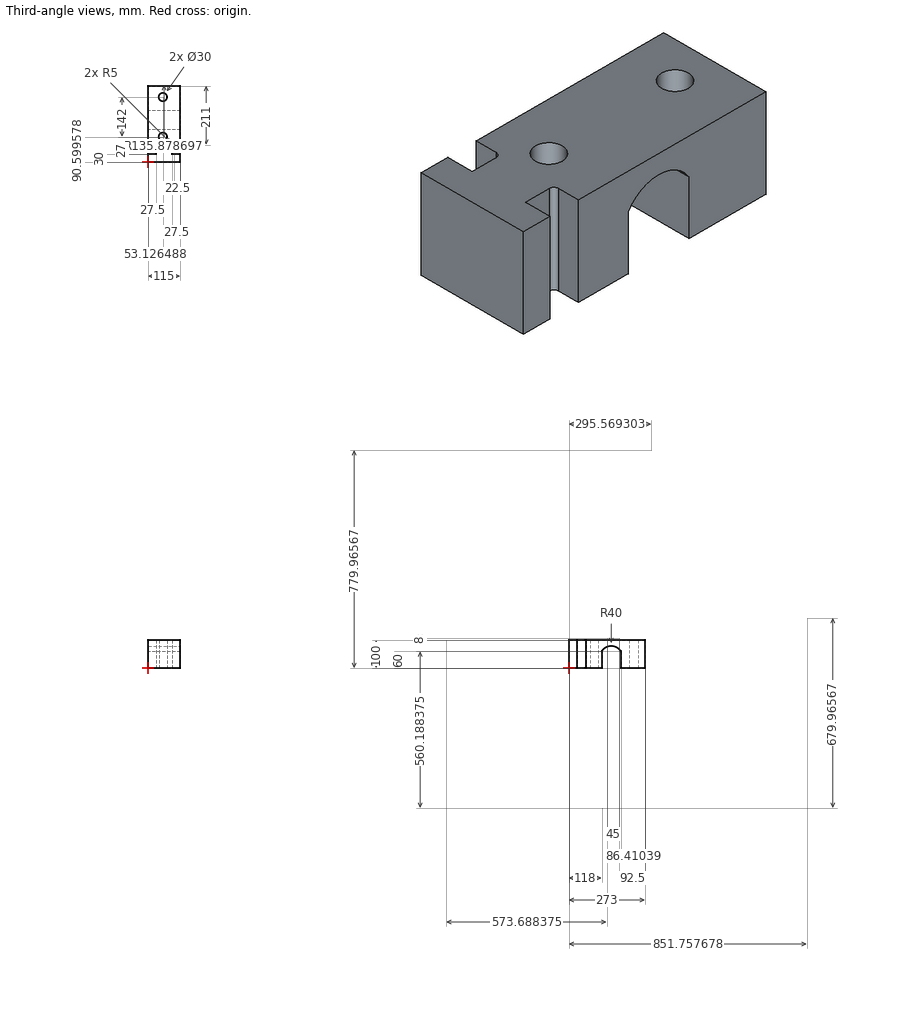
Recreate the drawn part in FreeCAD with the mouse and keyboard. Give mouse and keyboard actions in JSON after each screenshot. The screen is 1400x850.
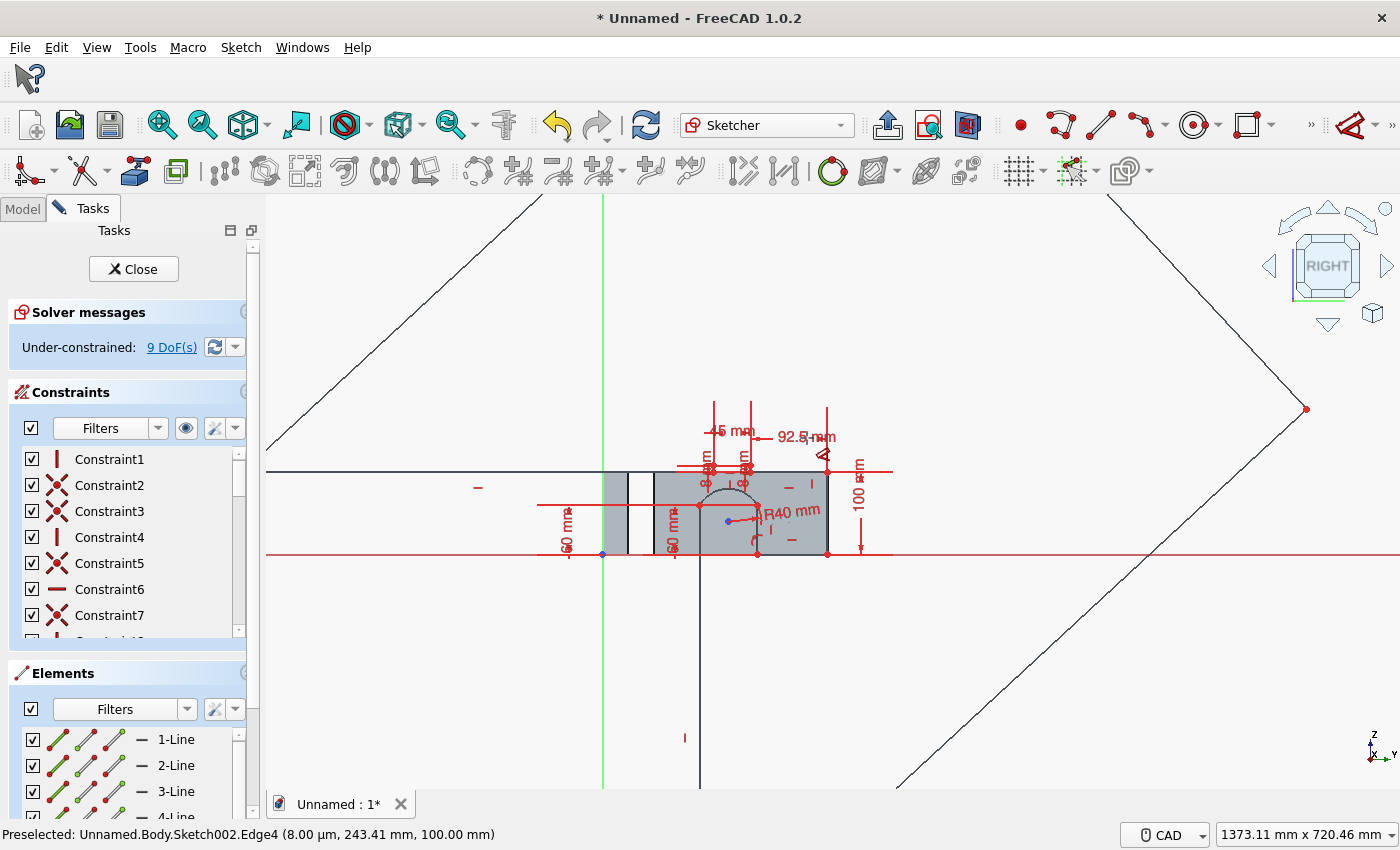
{"action": "left_click", "coordinate": [827, 555]}
{"action": "left_click", "coordinate": [715, 589]}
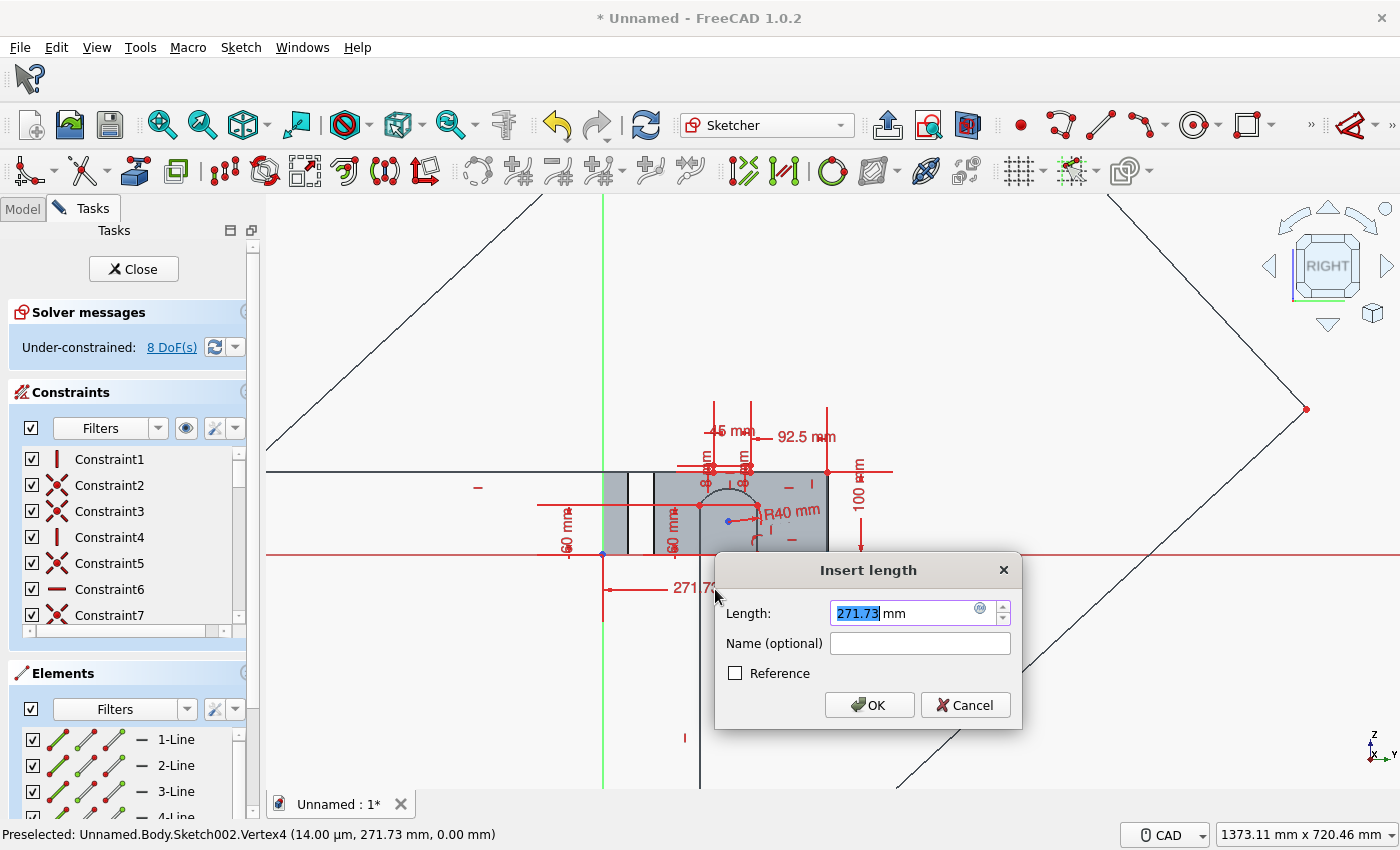
{"action": "type", "text": "273"}
{"action": "key", "text": "Return"}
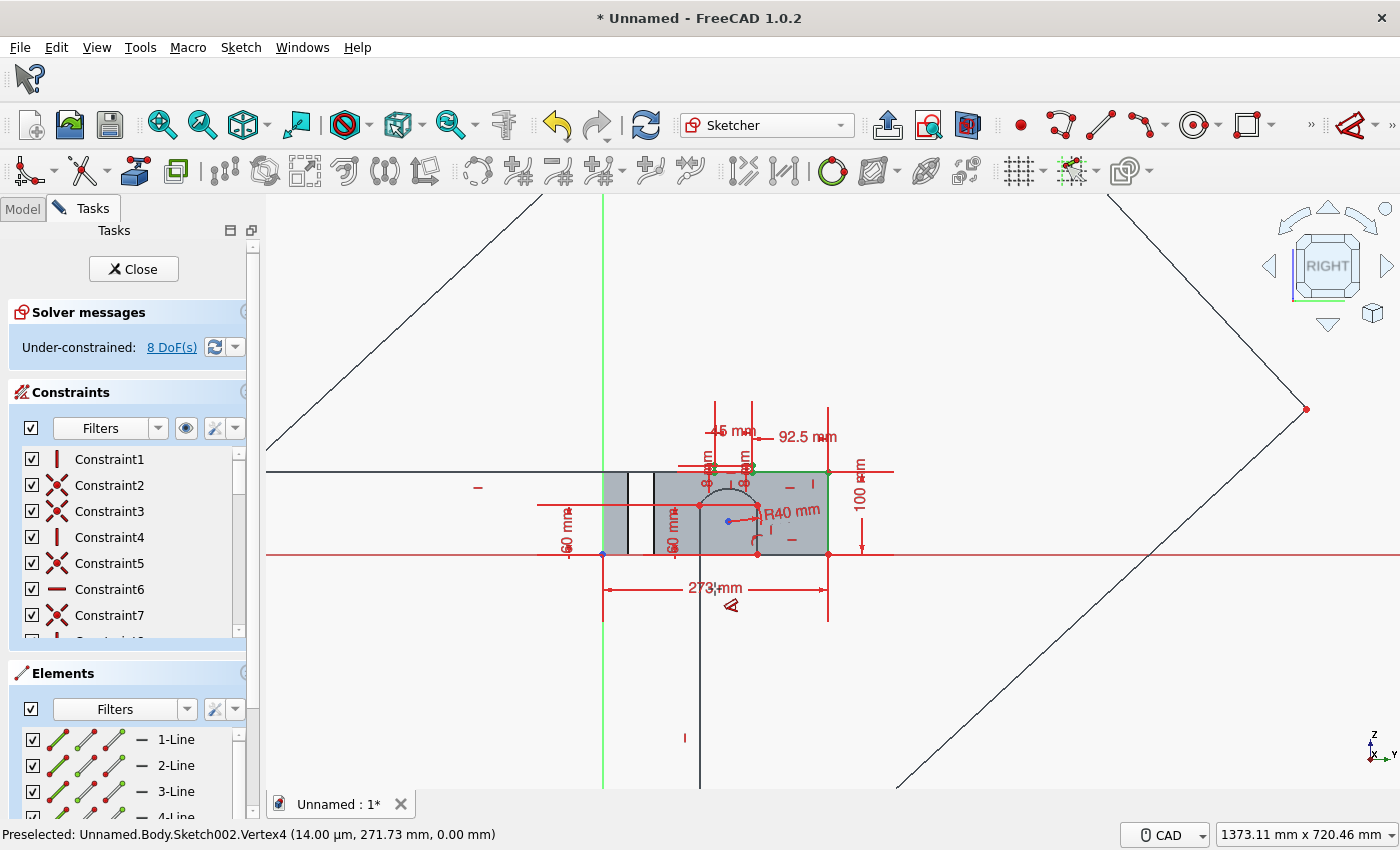
{"action": "scroll", "coordinate": [759, 522], "scroll_direction": "down", "scroll_amount": 5}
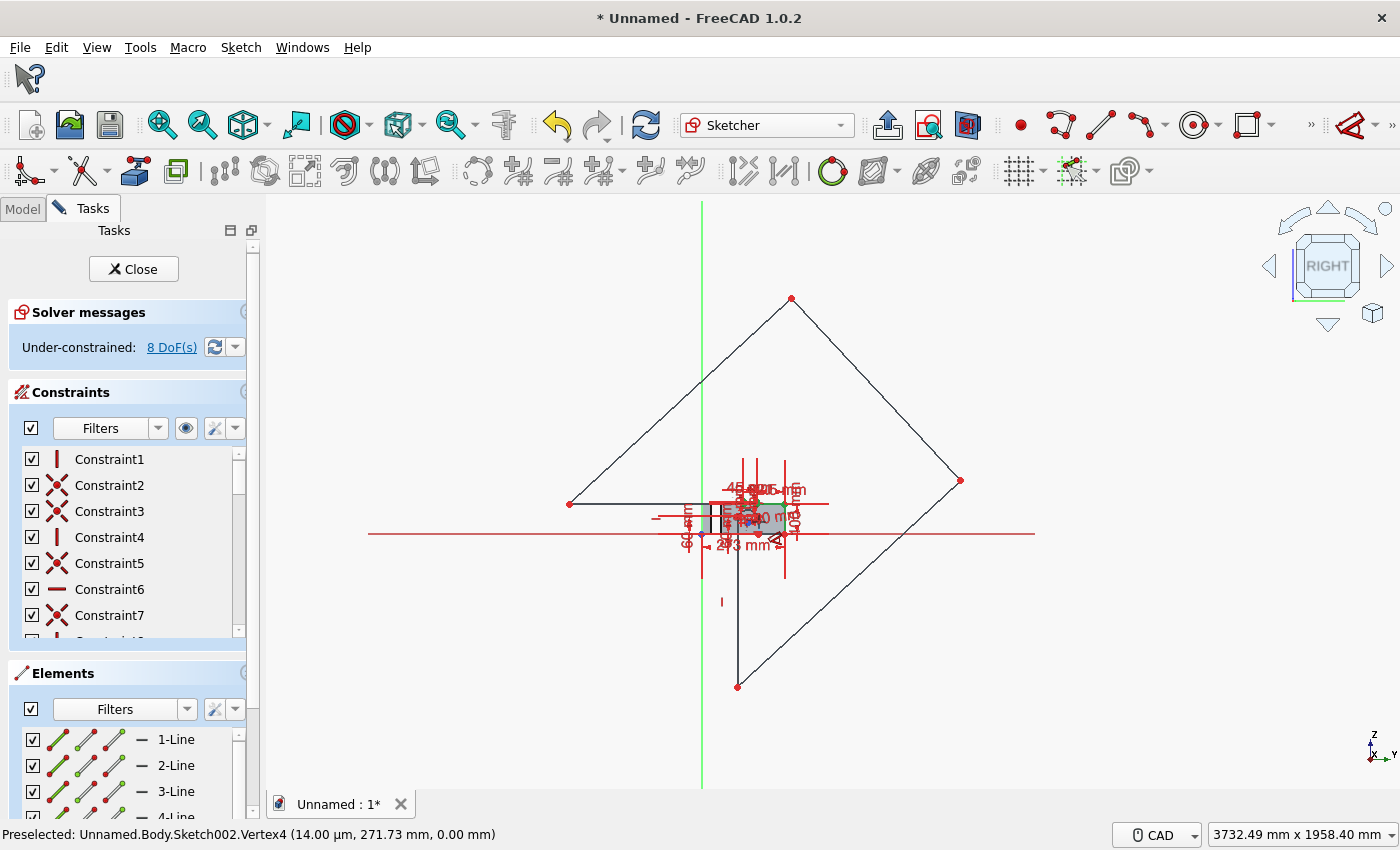
{"action": "left_click", "coordinate": [738, 687]}
{"action": "left_click", "coordinate": [720, 721]}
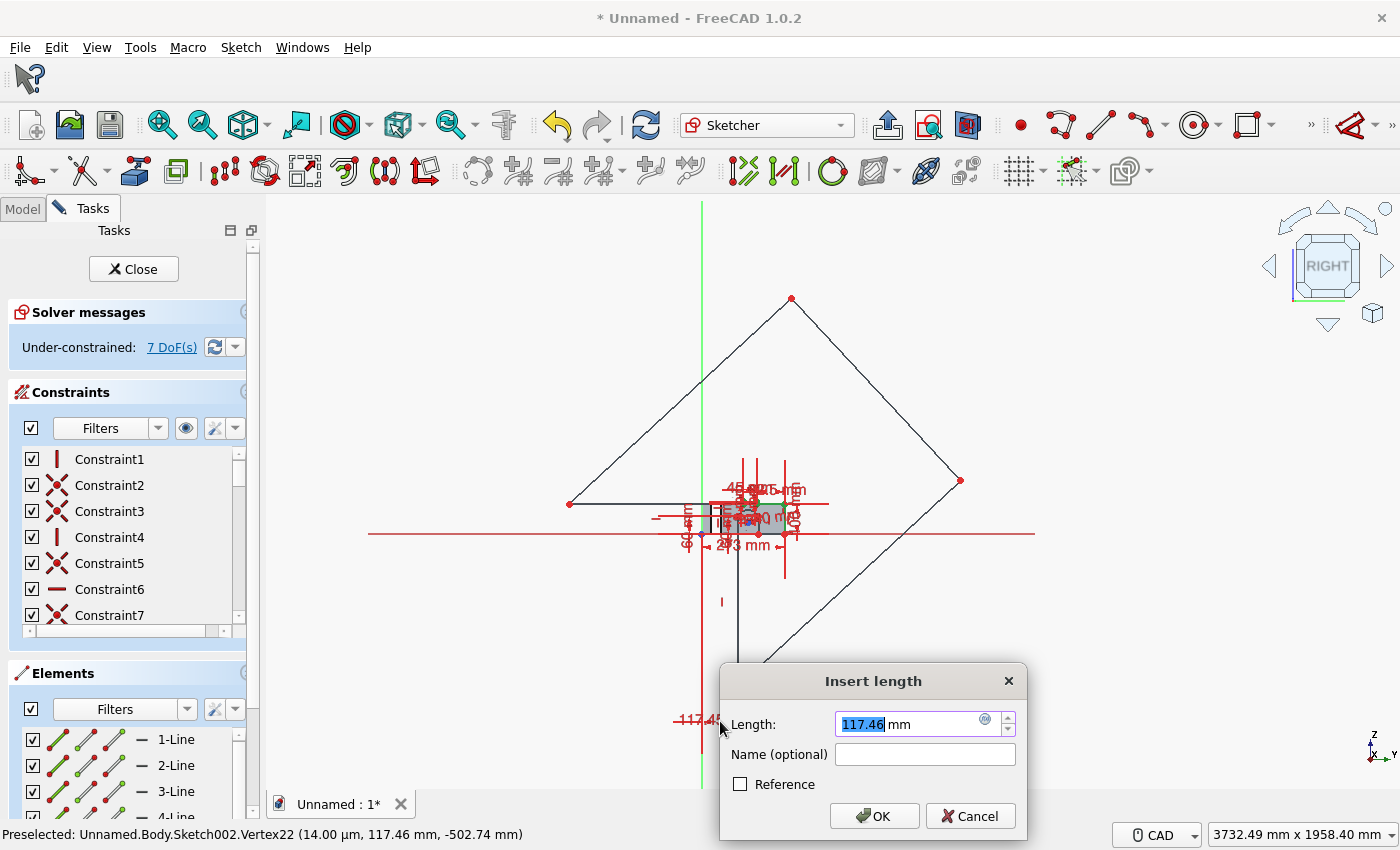
{"action": "type", "text": "118"}
{"action": "key", "text": "Return"}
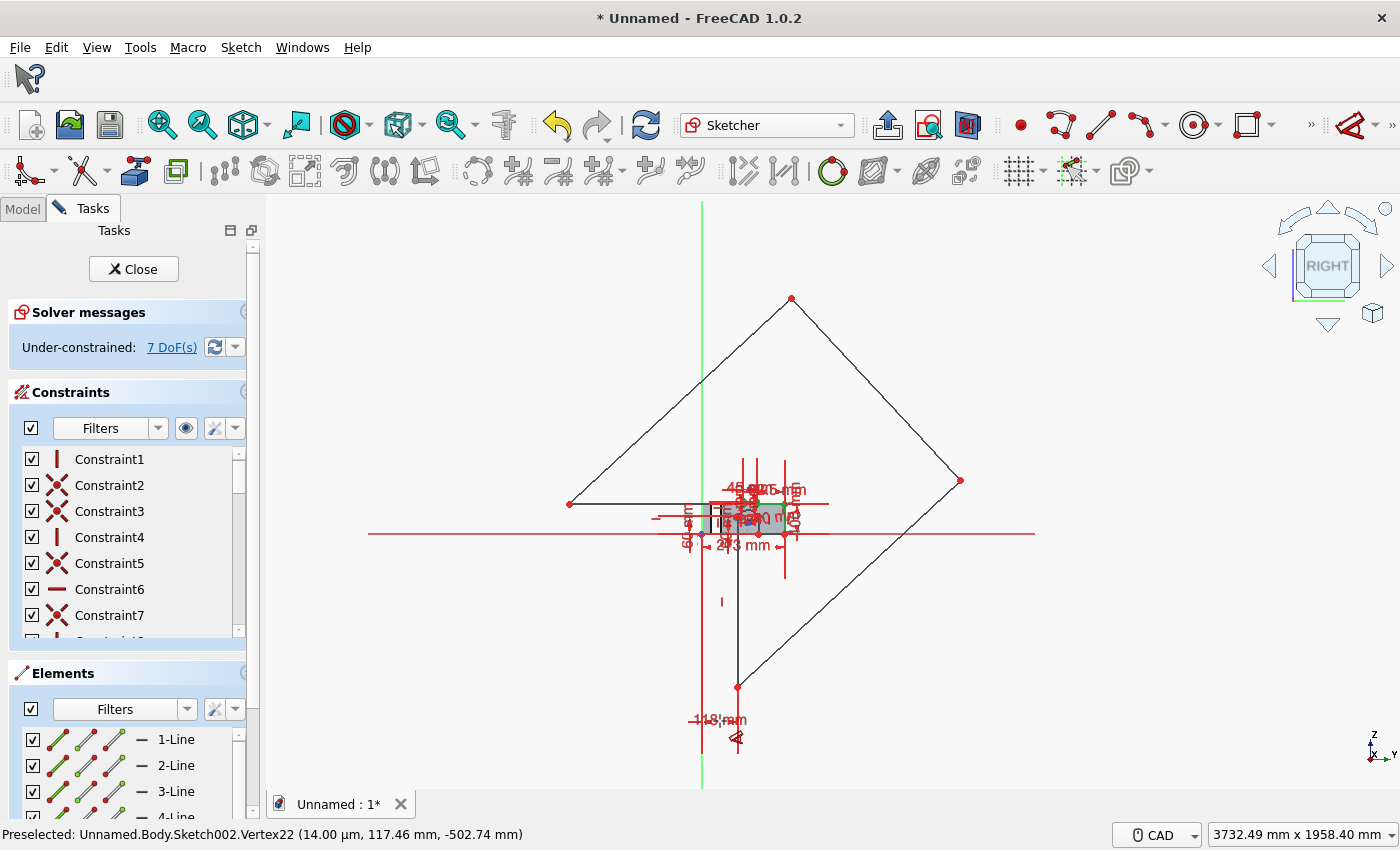
{"action": "scroll", "coordinate": [769, 534], "scroll_direction": "up", "scroll_amount": 3}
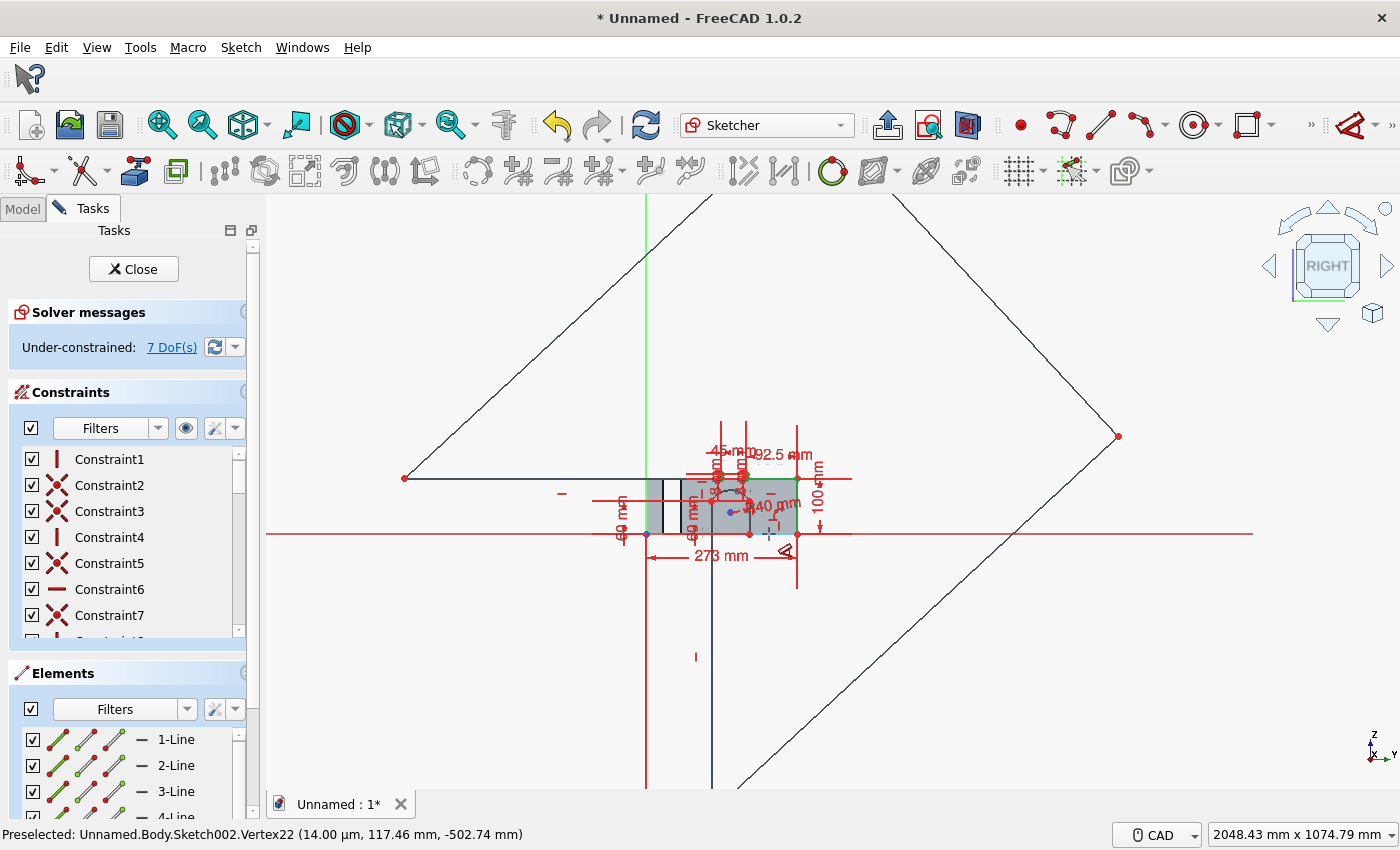
{"action": "left_click", "coordinate": [769, 534]}
{"action": "left_click", "coordinate": [774, 592]}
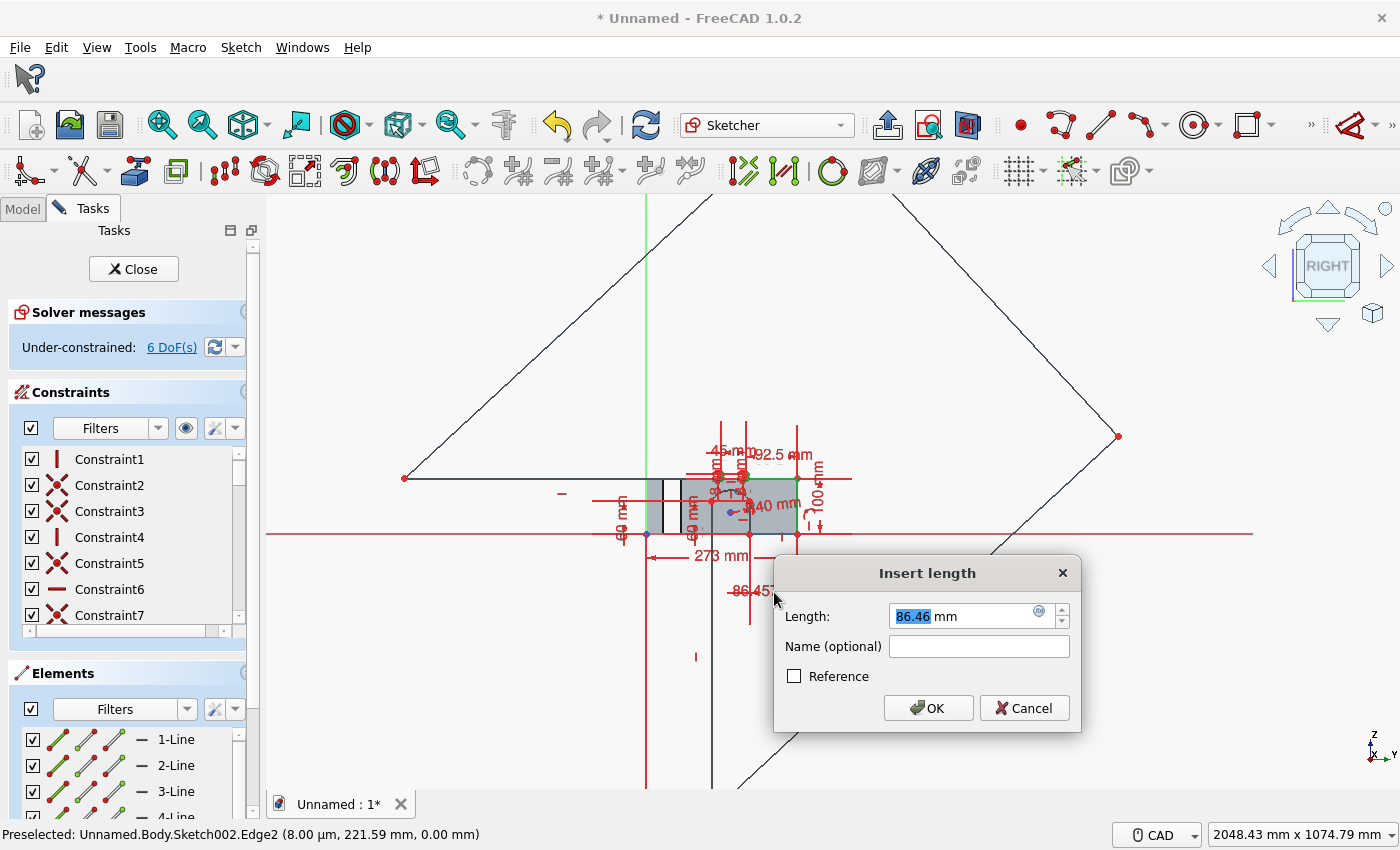
{"action": "type", "text": "86.41039"}
{"action": "key", "text": "Return"}